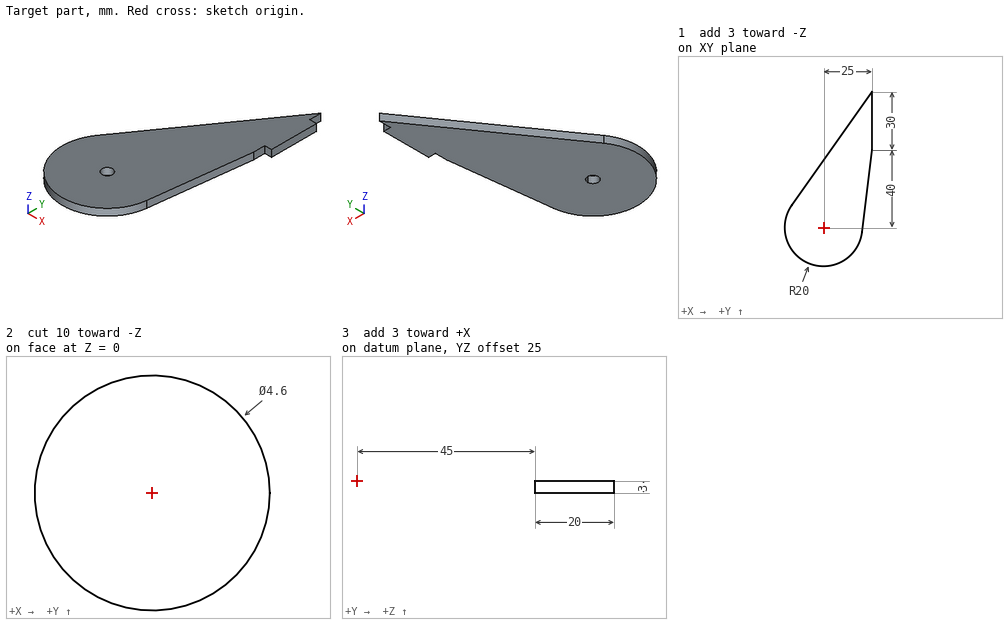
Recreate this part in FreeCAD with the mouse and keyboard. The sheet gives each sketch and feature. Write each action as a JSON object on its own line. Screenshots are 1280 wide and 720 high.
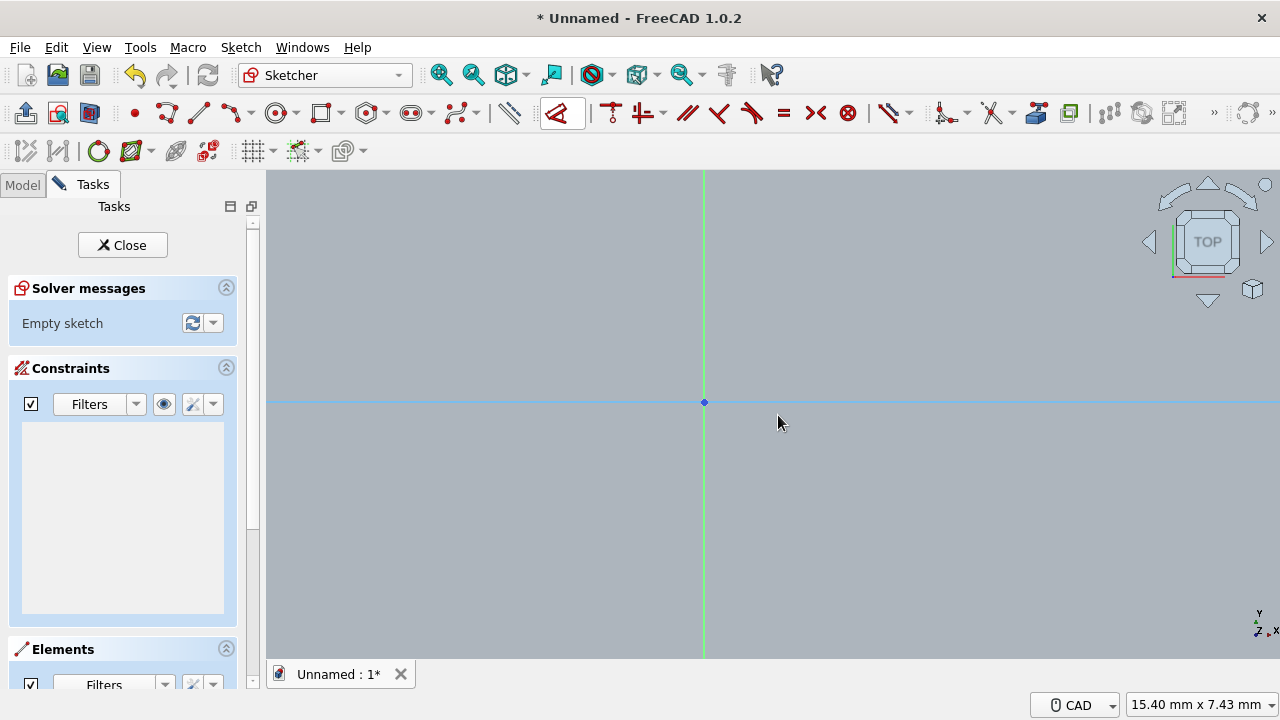
{"action": "left_click", "coordinate": [276, 114]}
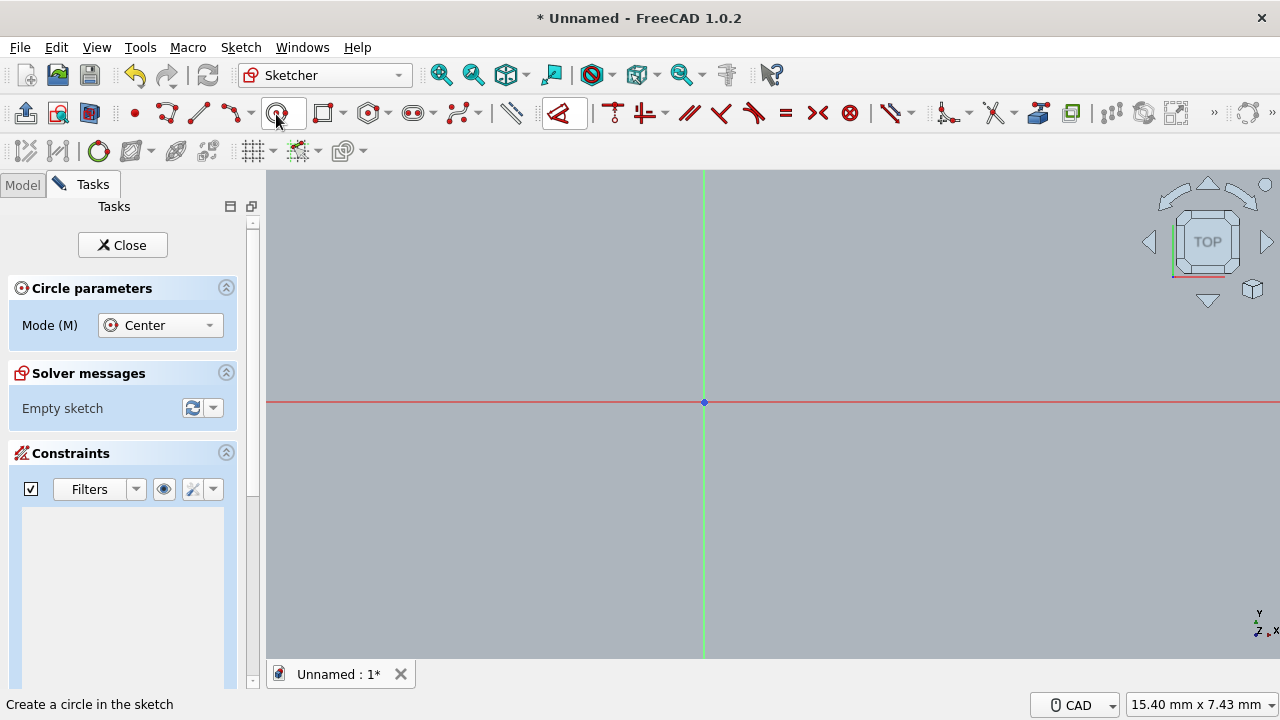
{"action": "left_click", "coordinate": [704, 402]}
{"action": "mouse_move", "coordinate": [811, 295]}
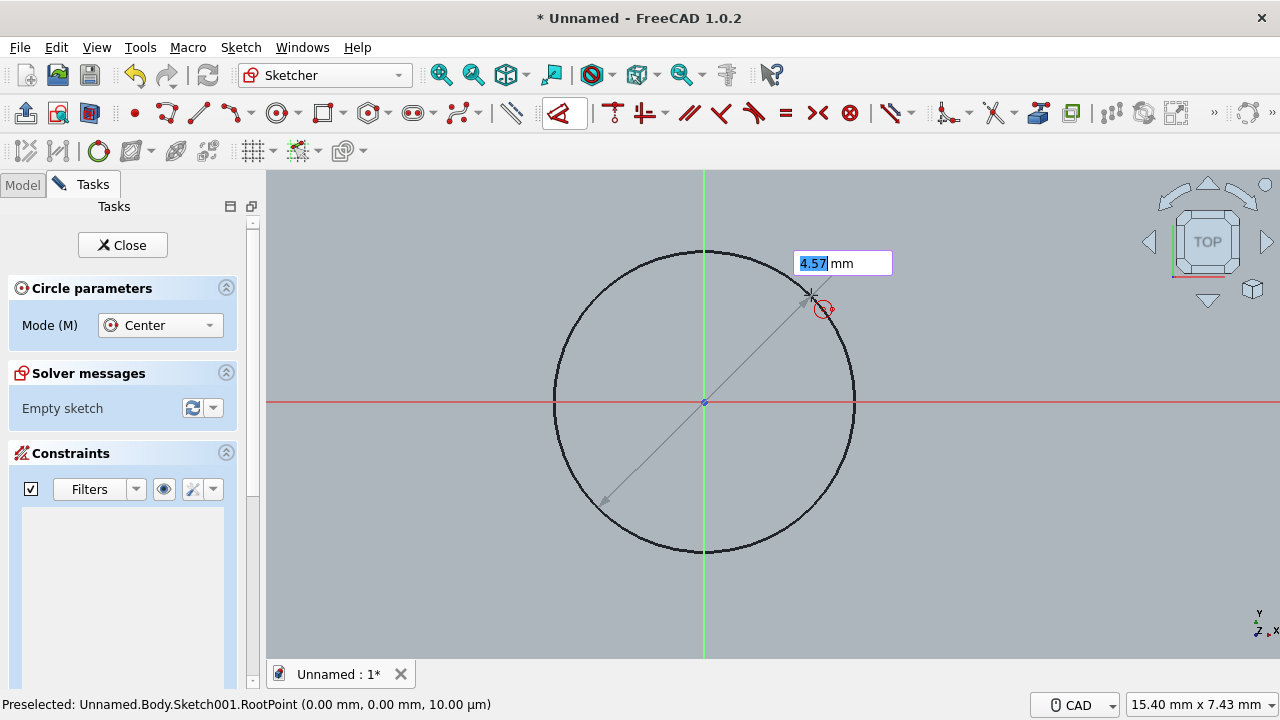
{"action": "type", "text": "4.6"}
{"action": "key", "text": "Return"}
{"action": "key", "text": "Escape"}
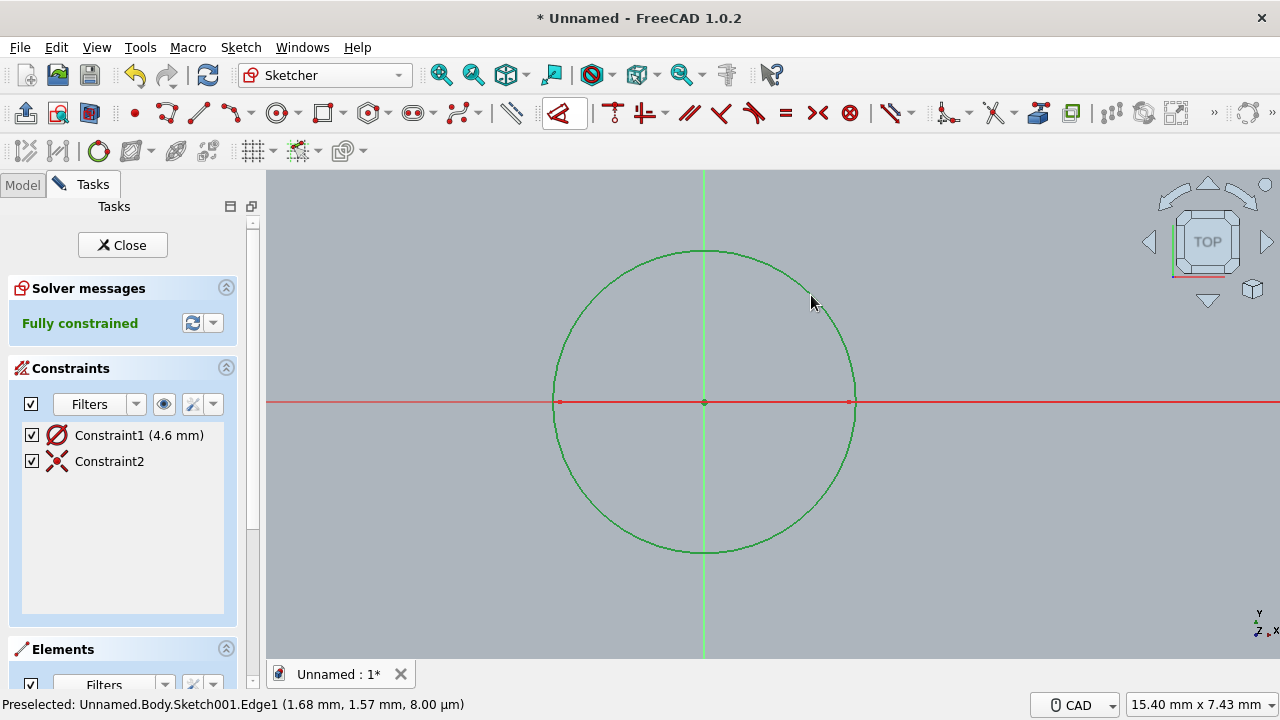
{"action": "left_click", "coordinate": [123, 245]}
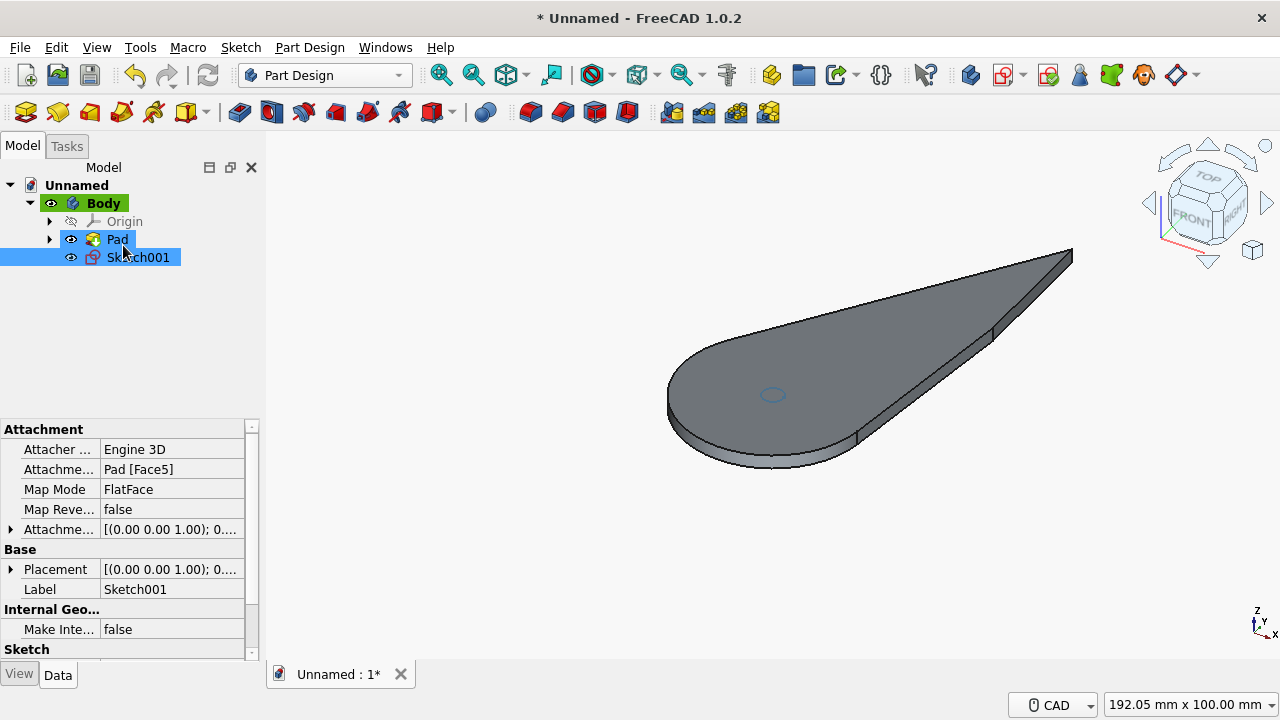
{"action": "left_click", "coordinate": [240, 112]}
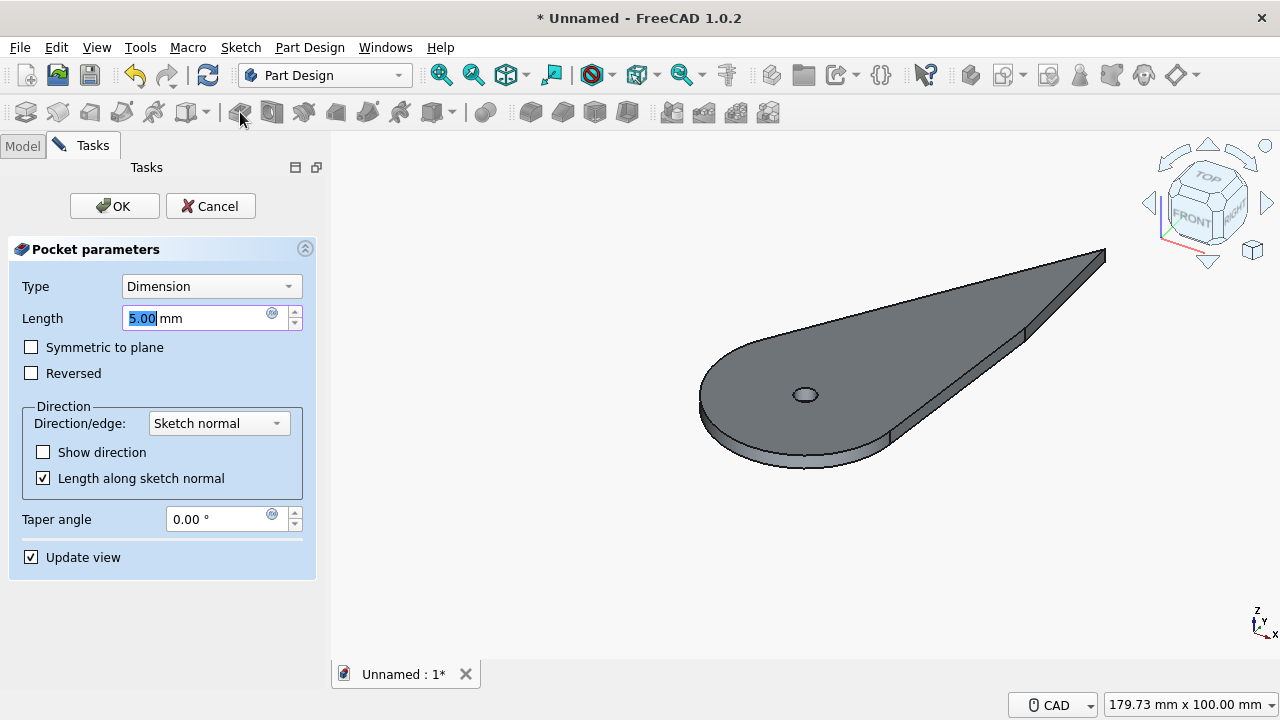
{"action": "type", "text": "10"}
{"action": "key", "text": "Tab"}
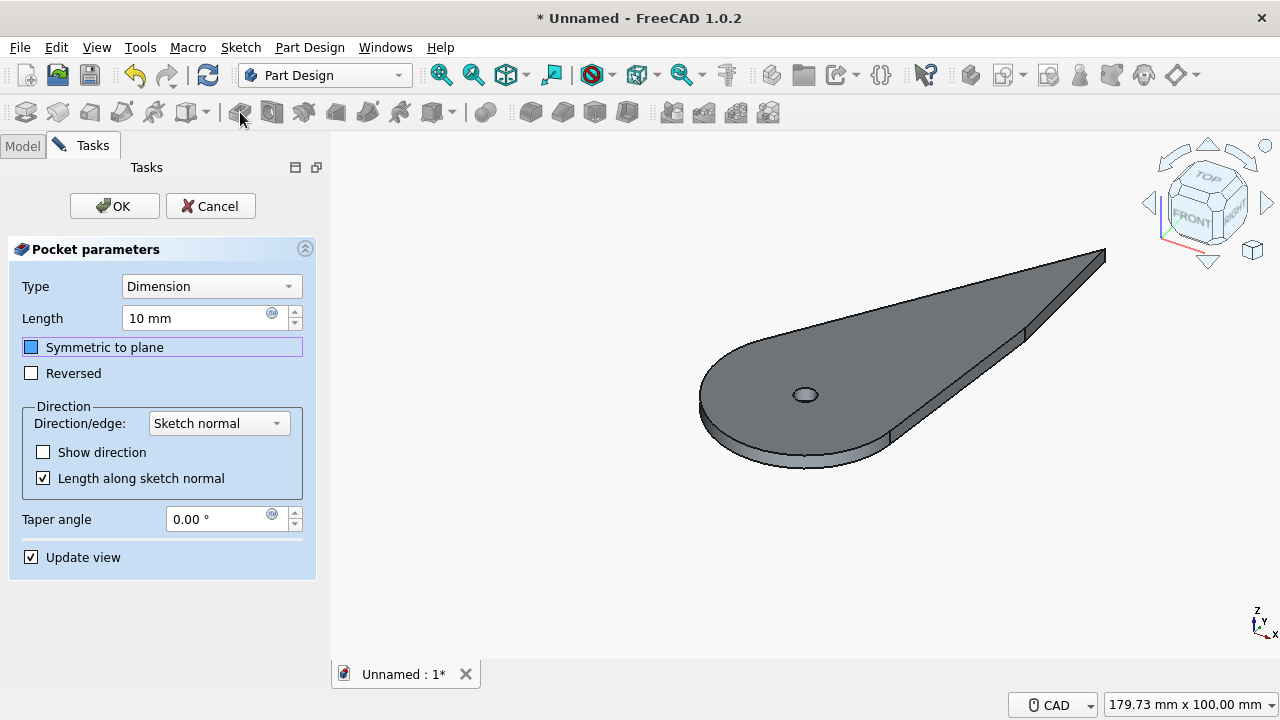
{"action": "left_click", "coordinate": [115, 206]}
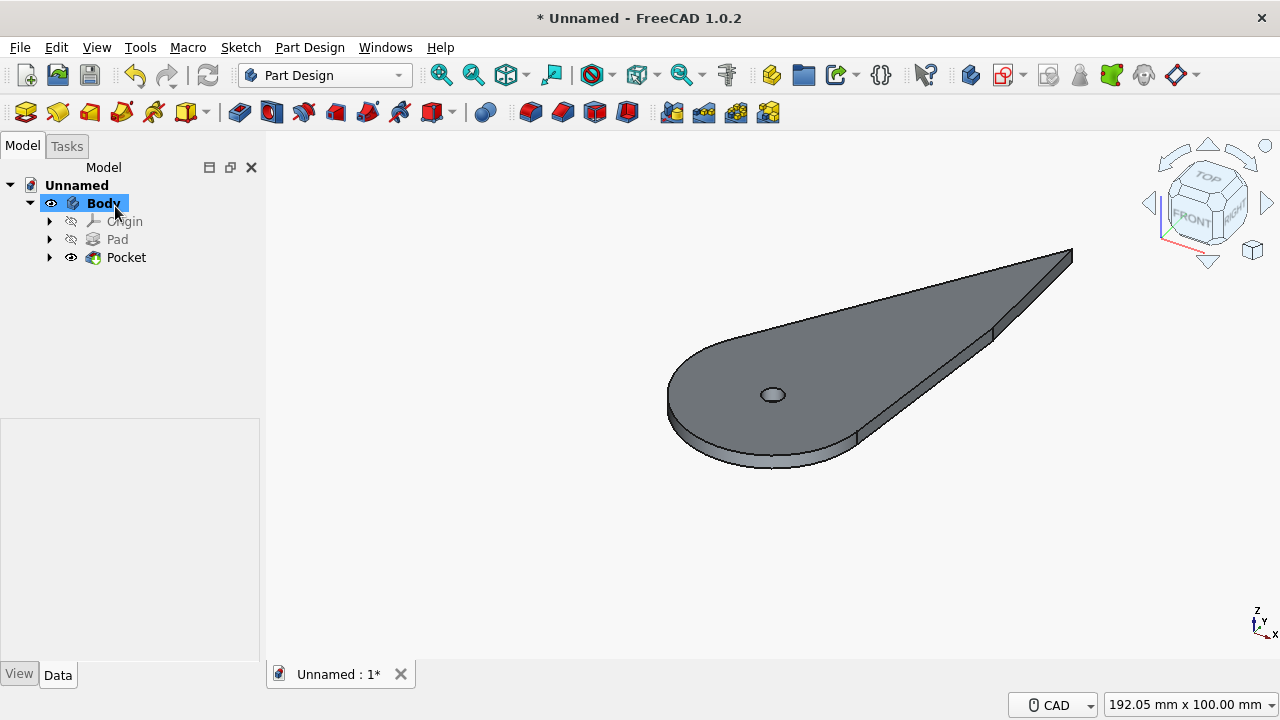
{"action": "key", "text": "0"}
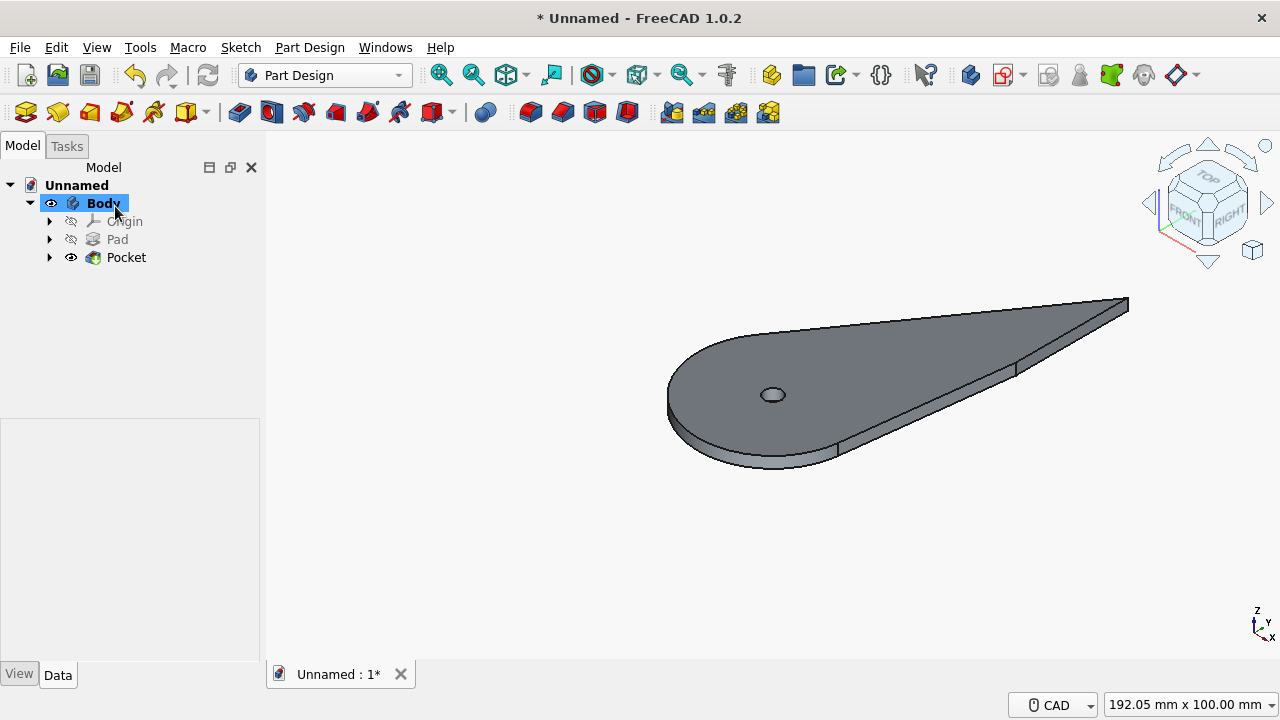
{"action": "key", "text": "3"}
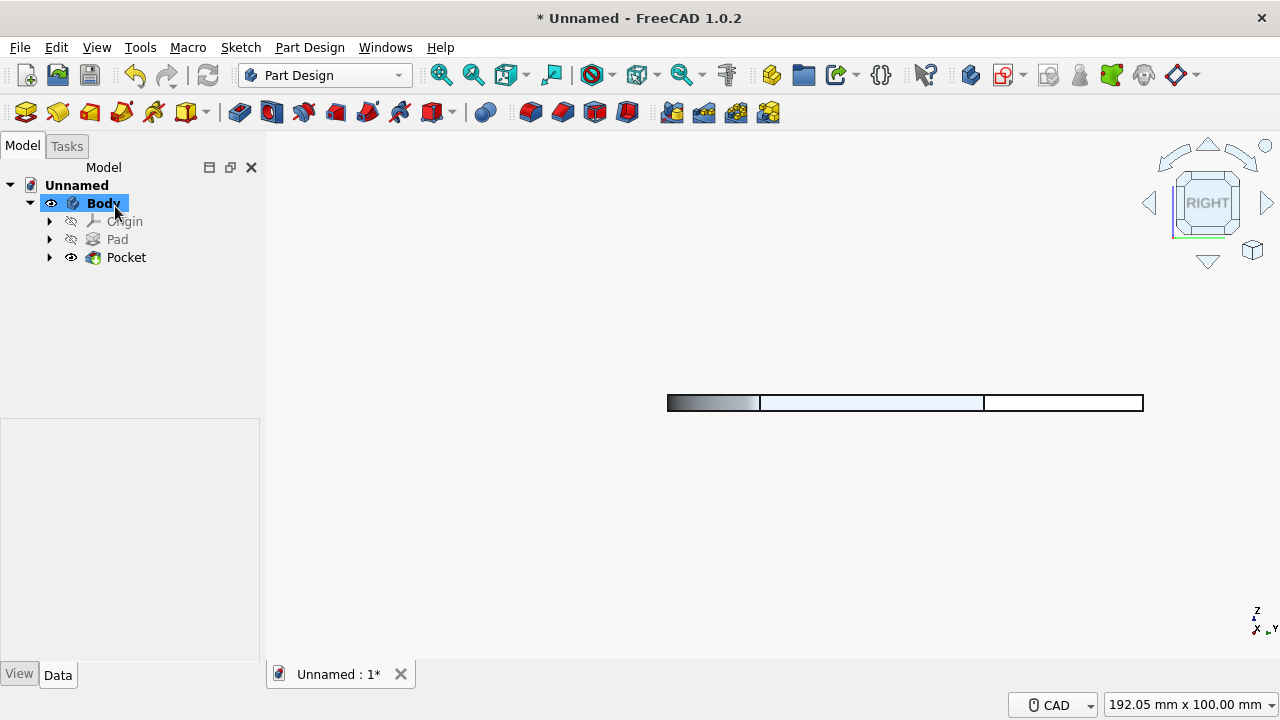
{"action": "key", "text": "2"}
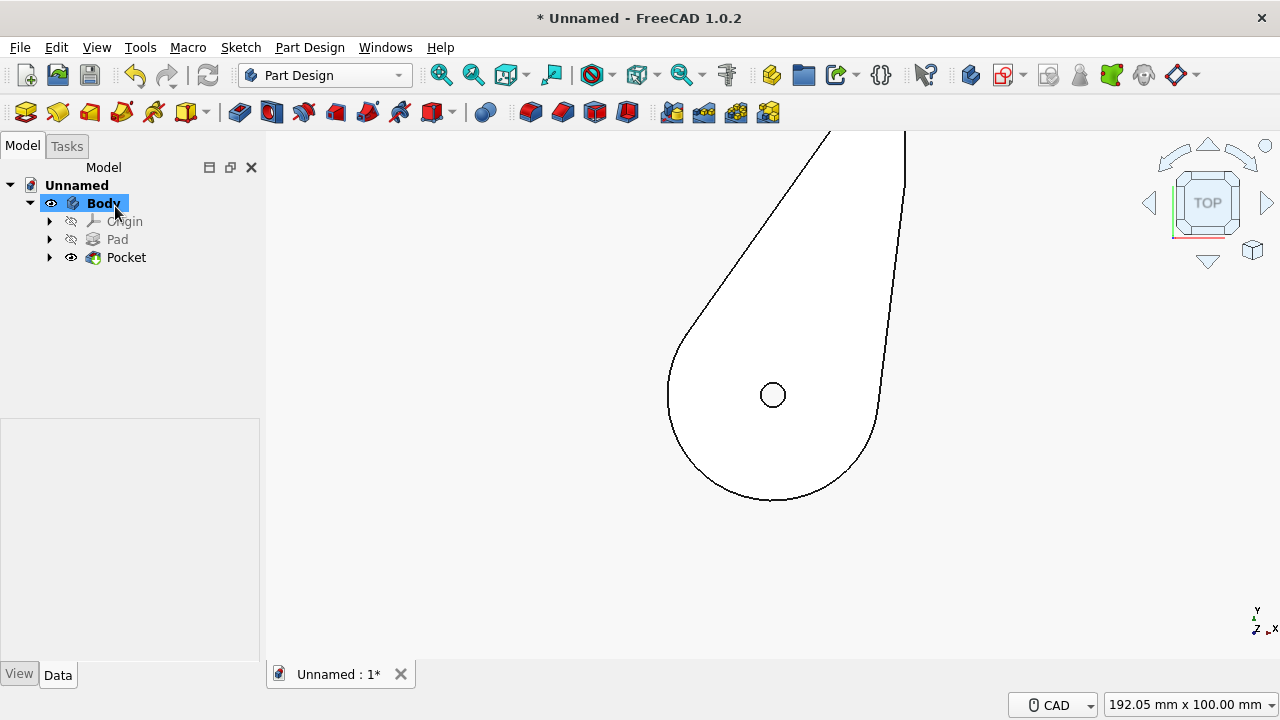
{"action": "key", "text": "v f"}